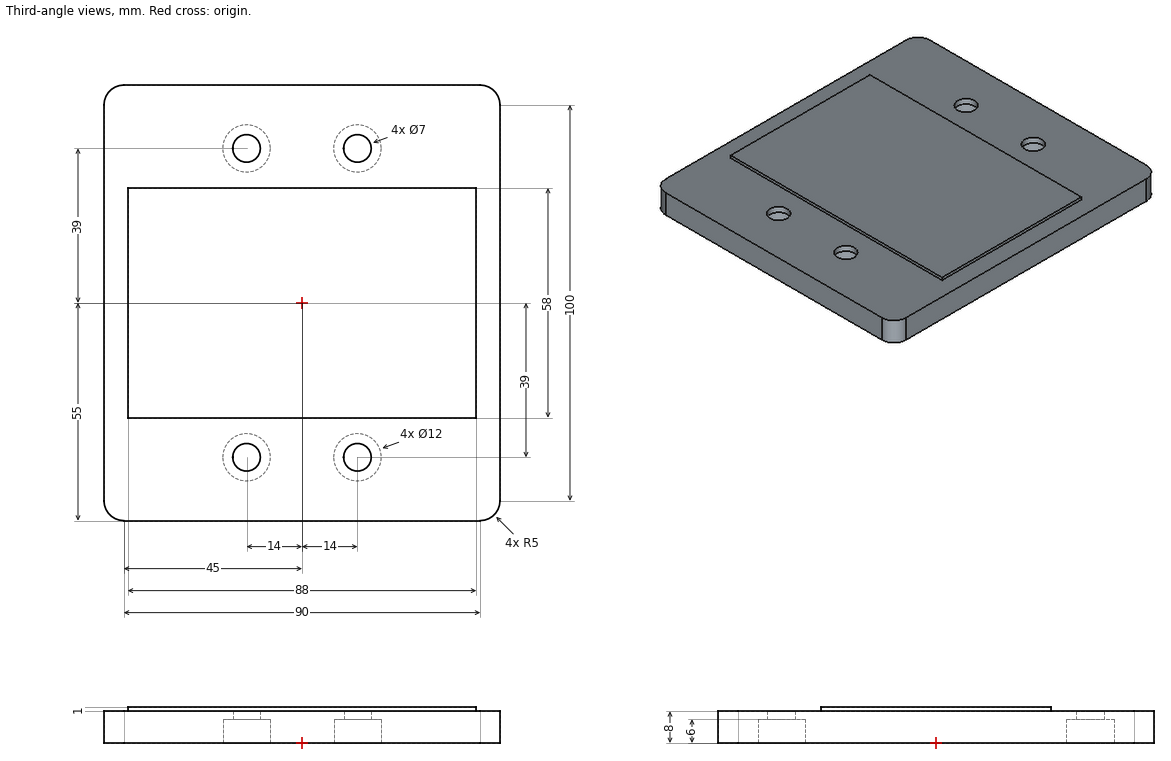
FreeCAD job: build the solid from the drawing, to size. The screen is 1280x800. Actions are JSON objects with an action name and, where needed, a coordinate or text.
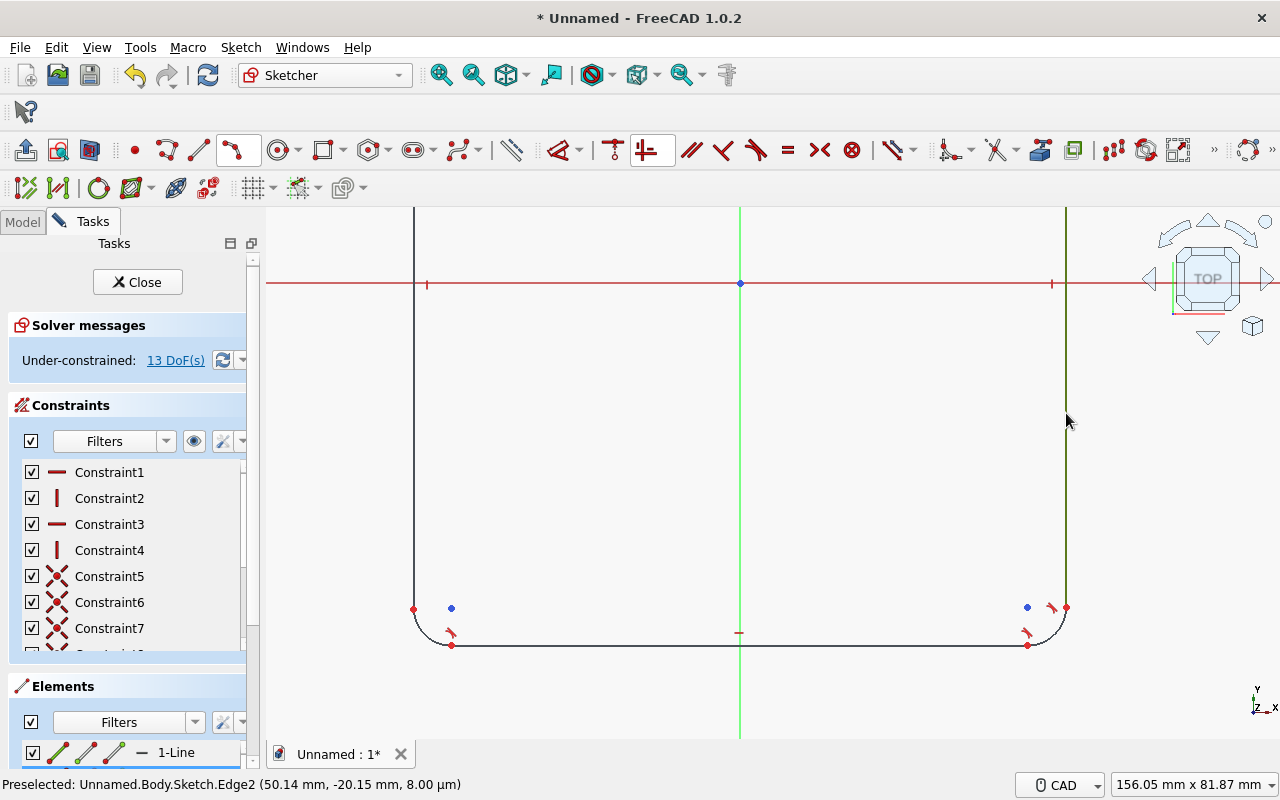
{"action": "scroll", "coordinate": [675, 628], "scroll_direction": "down", "scroll_amount": 4}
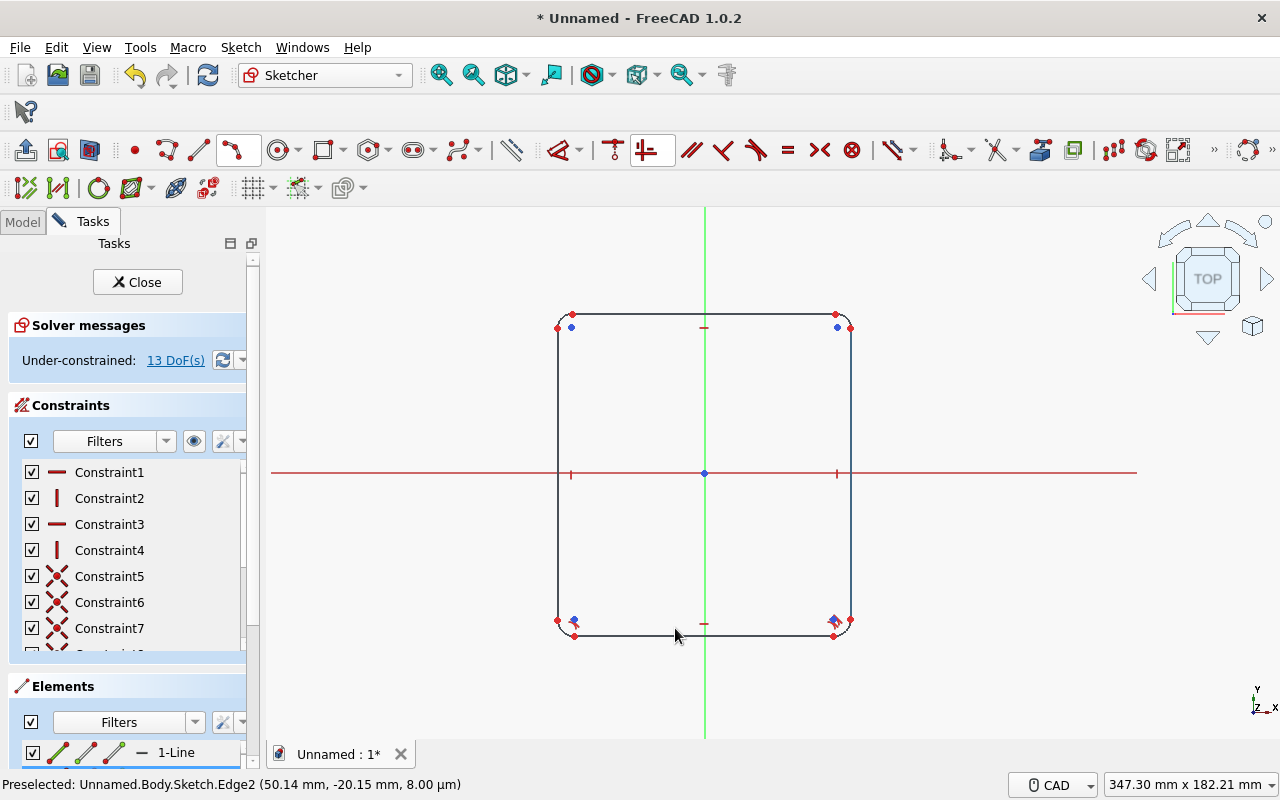
{"action": "scroll", "coordinate": [849, 322], "scroll_direction": "up", "scroll_amount": 4}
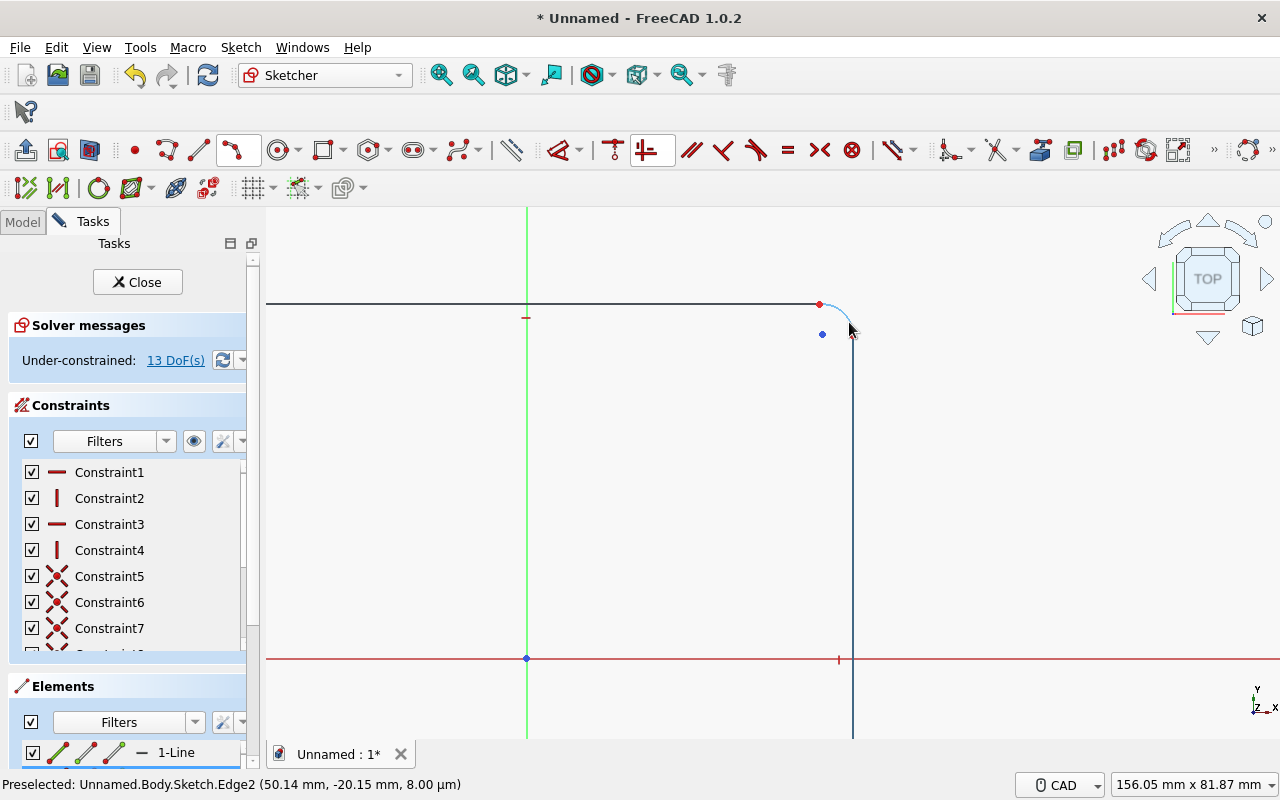
{"action": "left_click", "coordinate": [849, 321]}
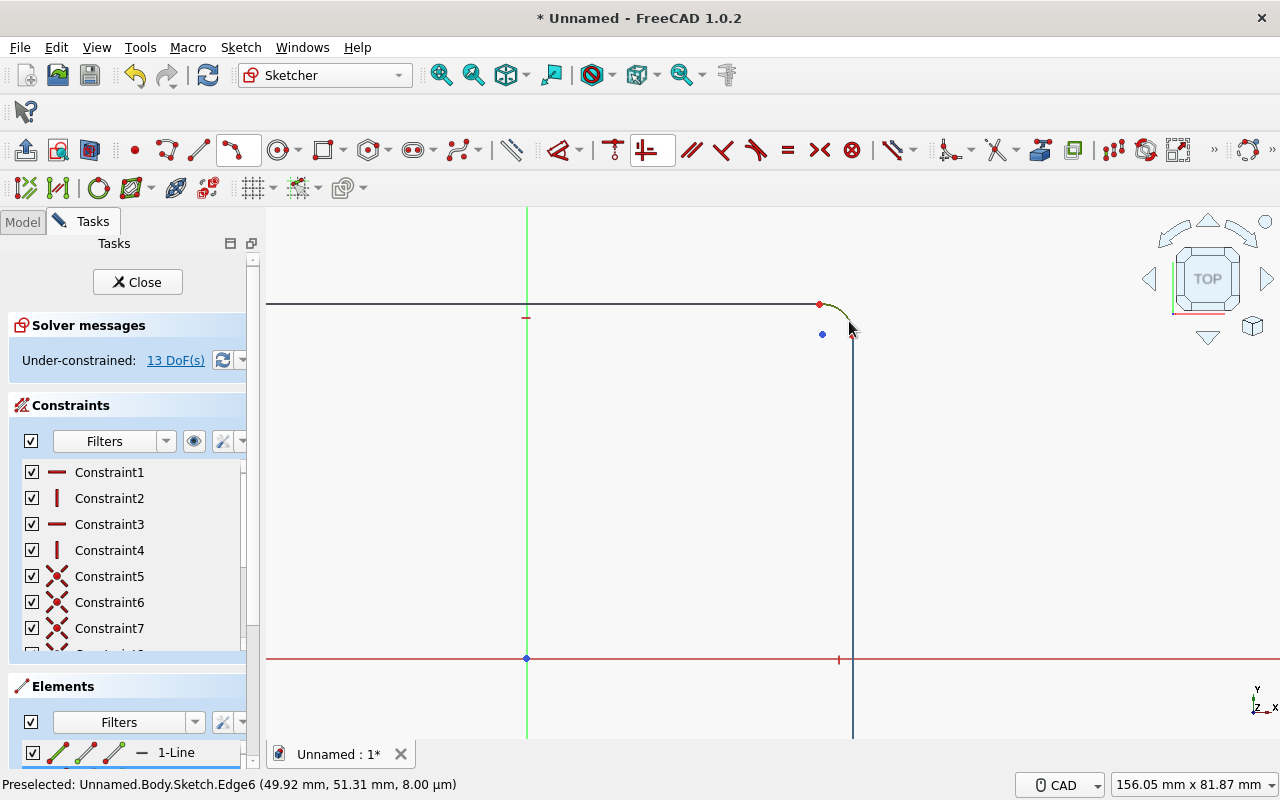
{"action": "key", "text": "t"}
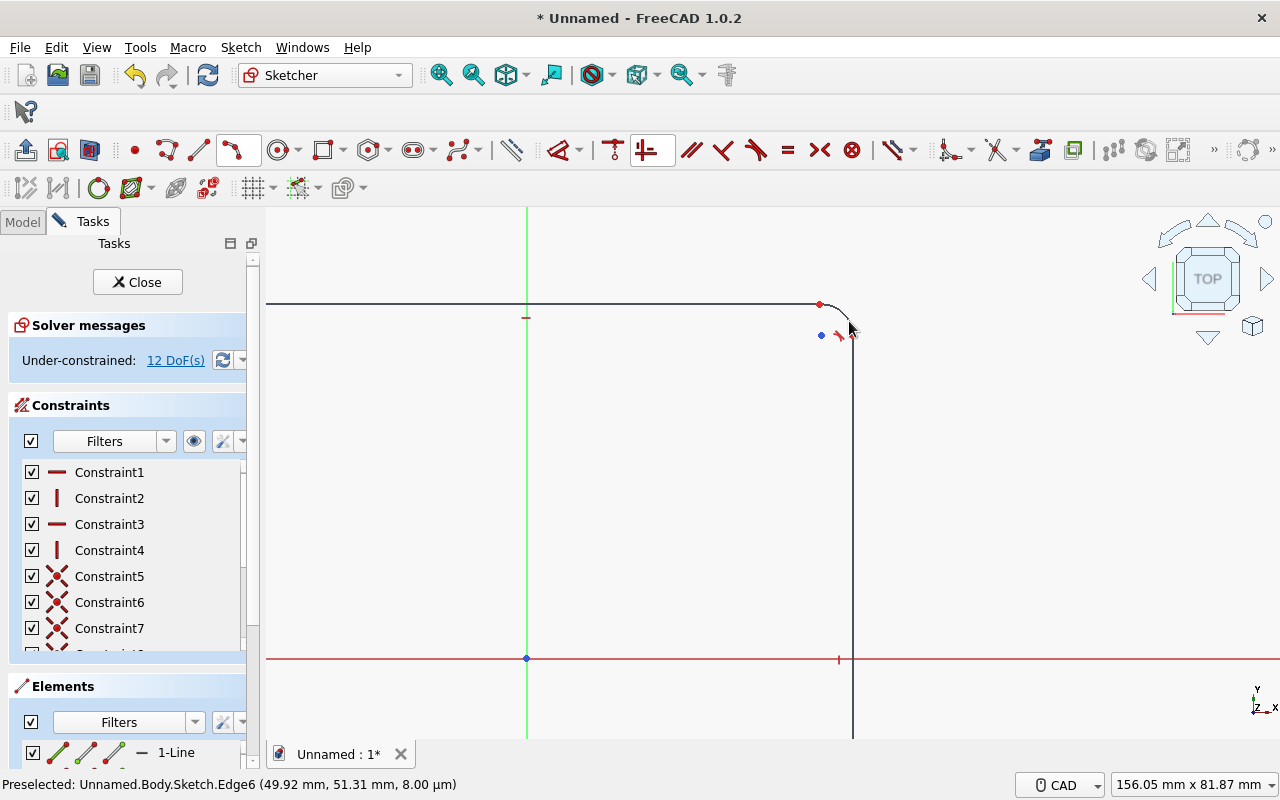
{"action": "left_click", "coordinate": [644, 304]}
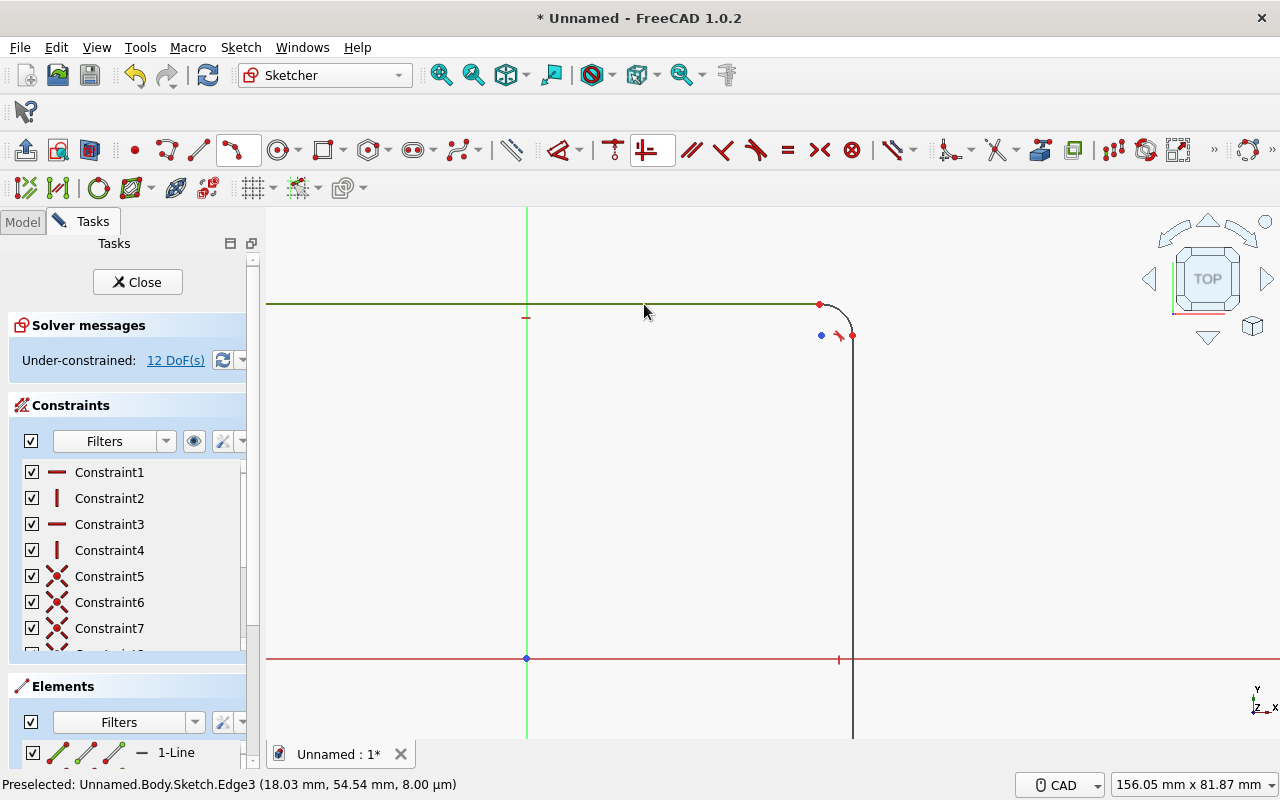
{"action": "left_click", "coordinate": [849, 321]}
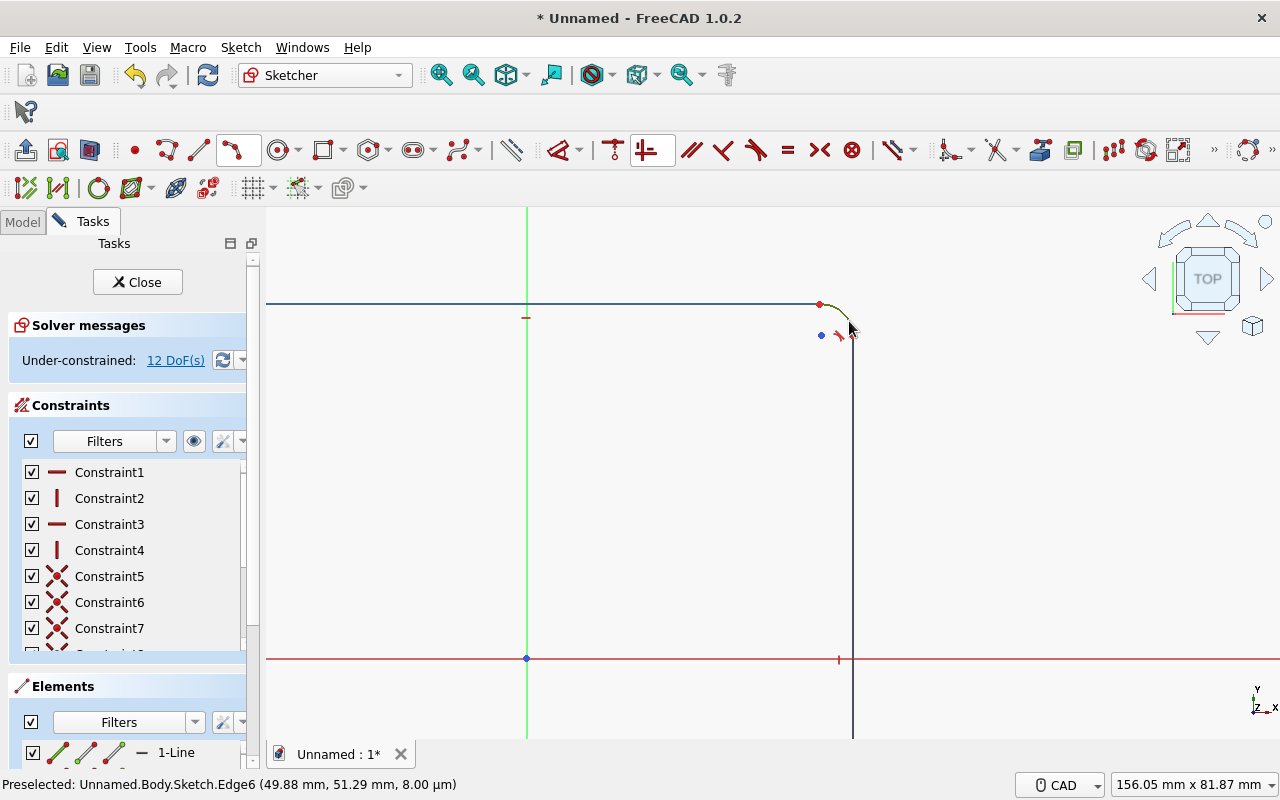
{"action": "key", "text": "t"}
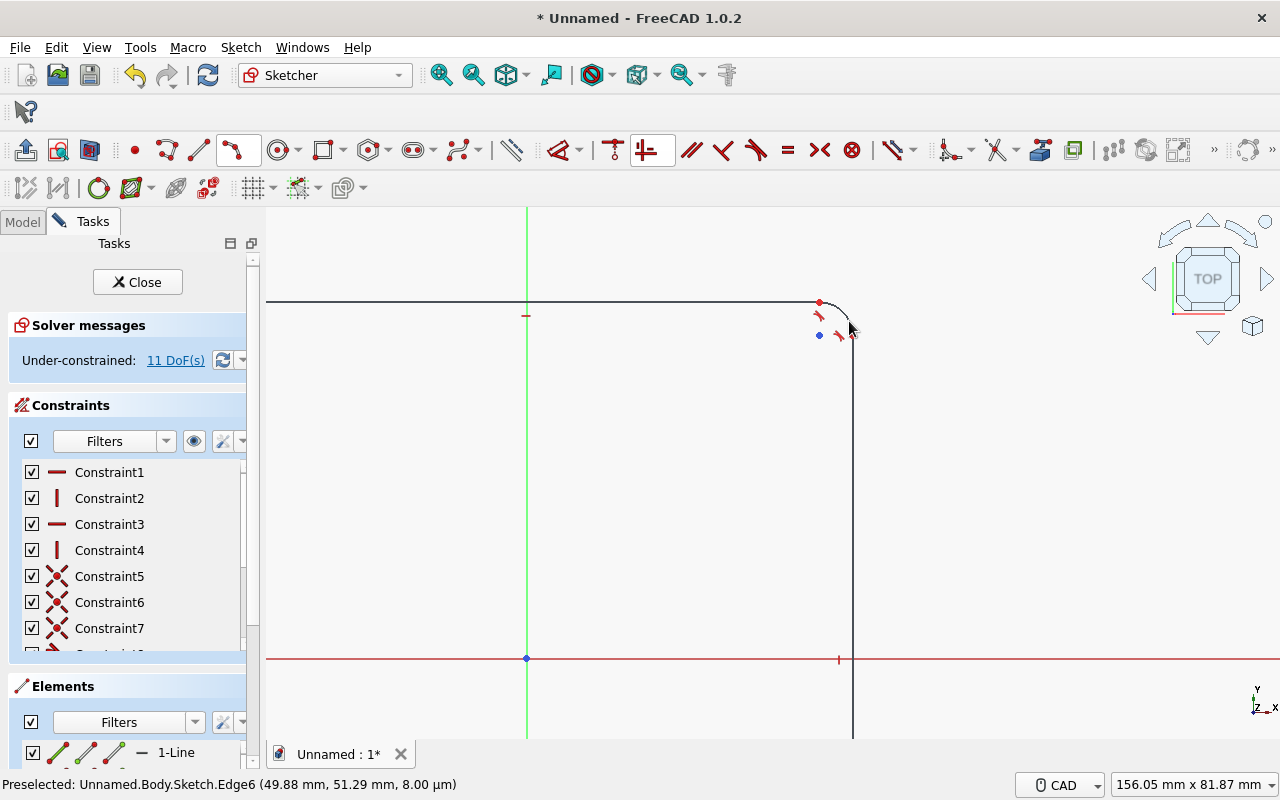
{"action": "left_click", "coordinate": [644, 302]}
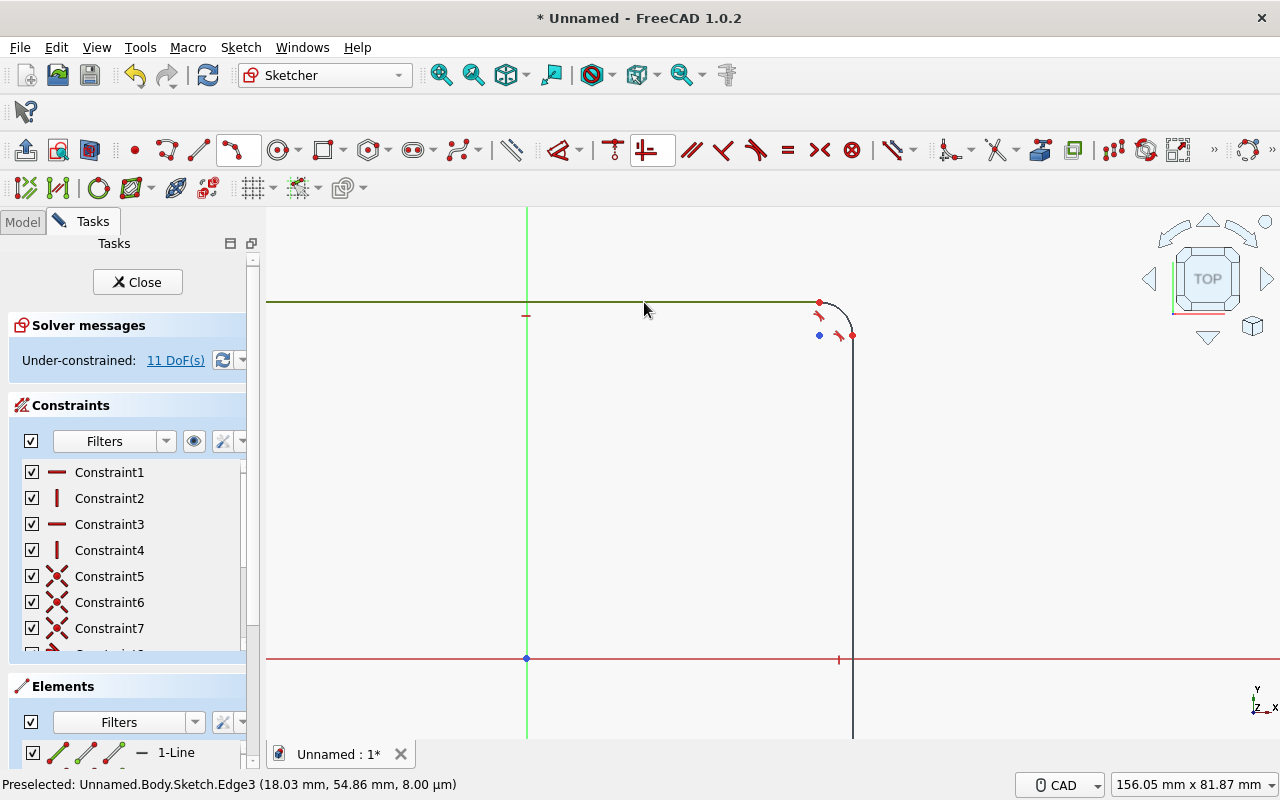
{"action": "scroll", "coordinate": [849, 321], "scroll_direction": "down", "scroll_amount": 4}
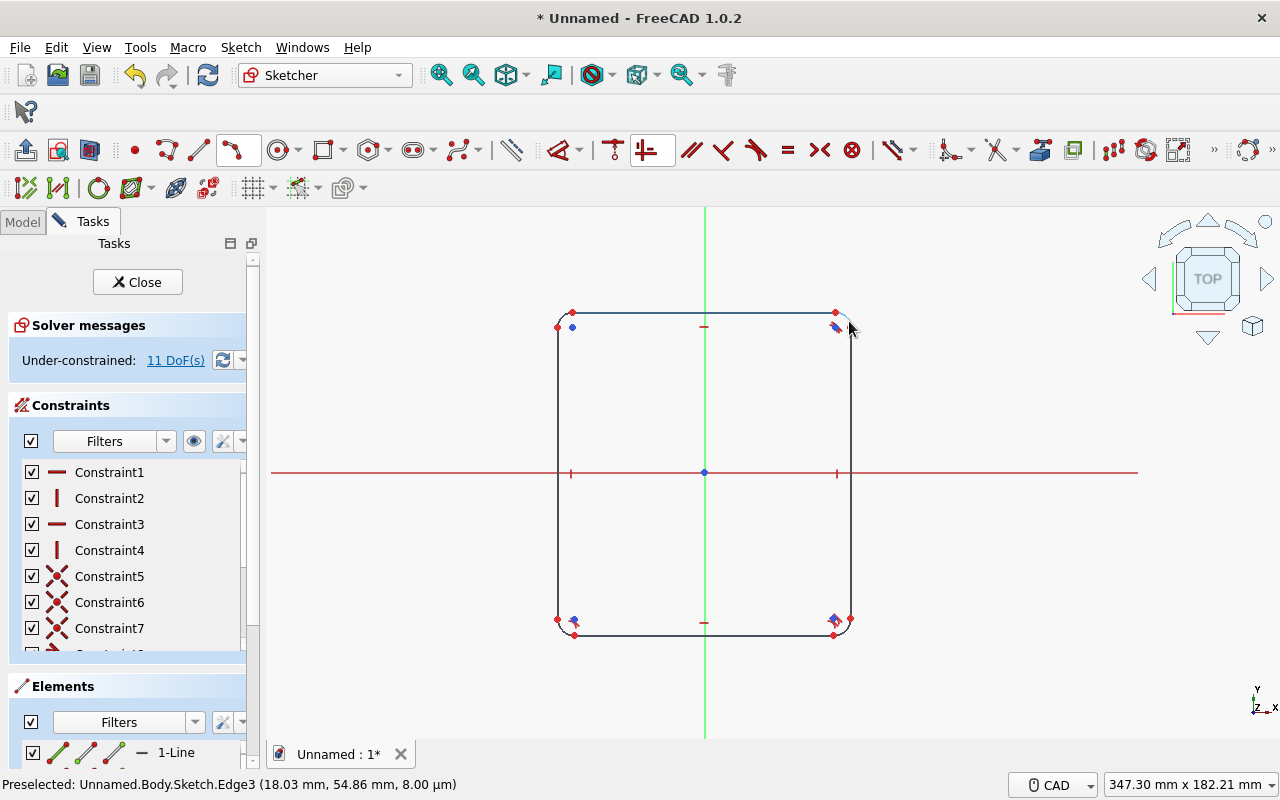
{"action": "scroll", "coordinate": [566, 314], "scroll_direction": "up", "scroll_amount": 4}